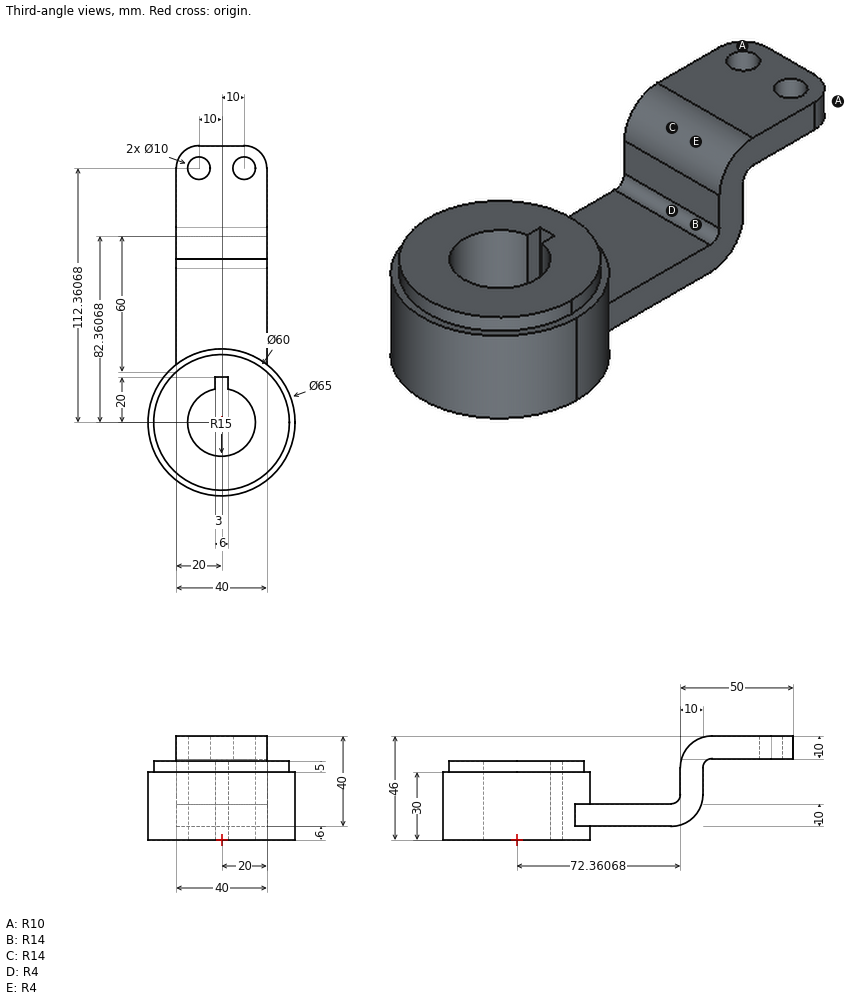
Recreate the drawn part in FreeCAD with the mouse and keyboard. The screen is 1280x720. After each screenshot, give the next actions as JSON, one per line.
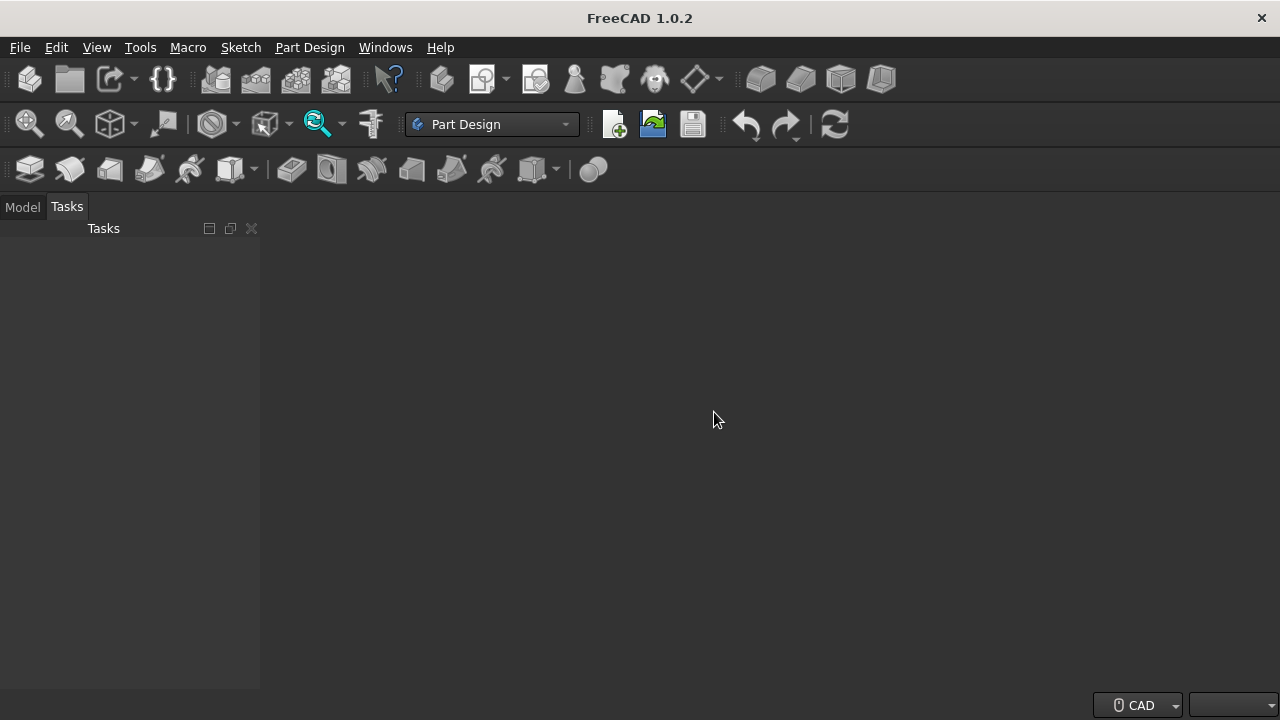
{"action": "key", "text": "ctrl+n"}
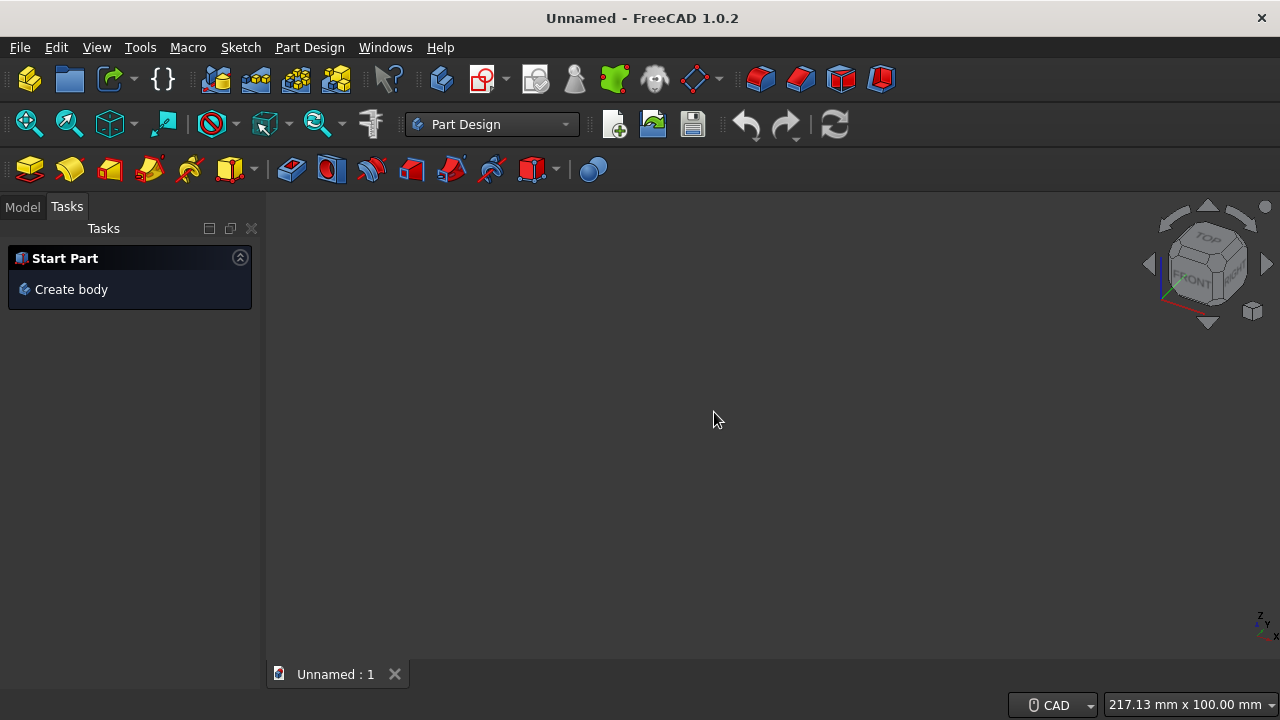
{"action": "left_click", "coordinate": [482, 80]}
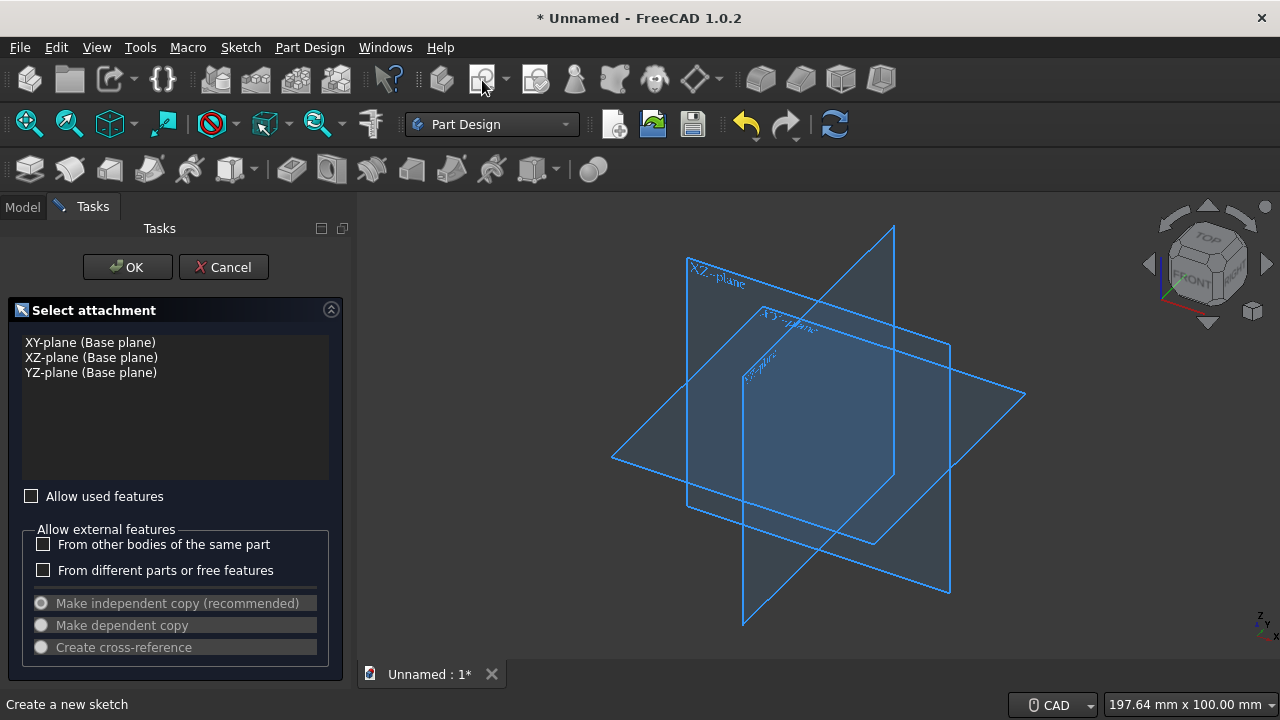
{"action": "left_click", "coordinate": [82, 342]}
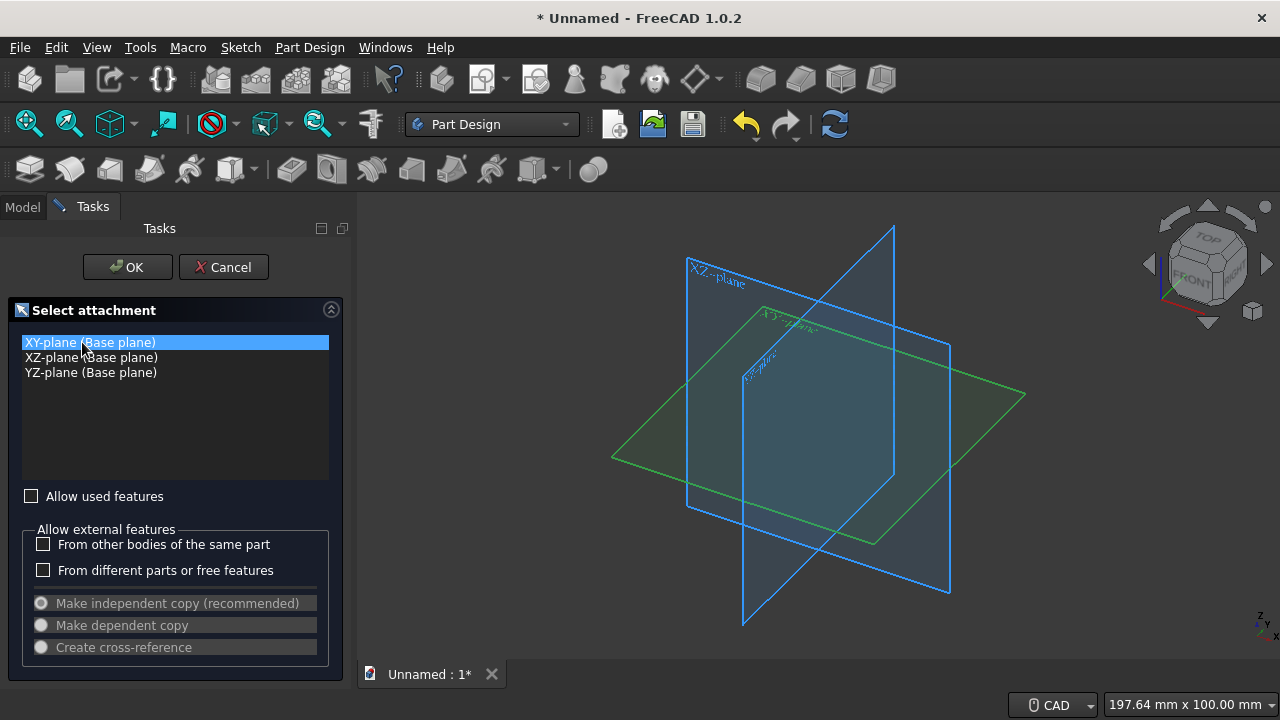
{"action": "left_click", "coordinate": [128, 267]}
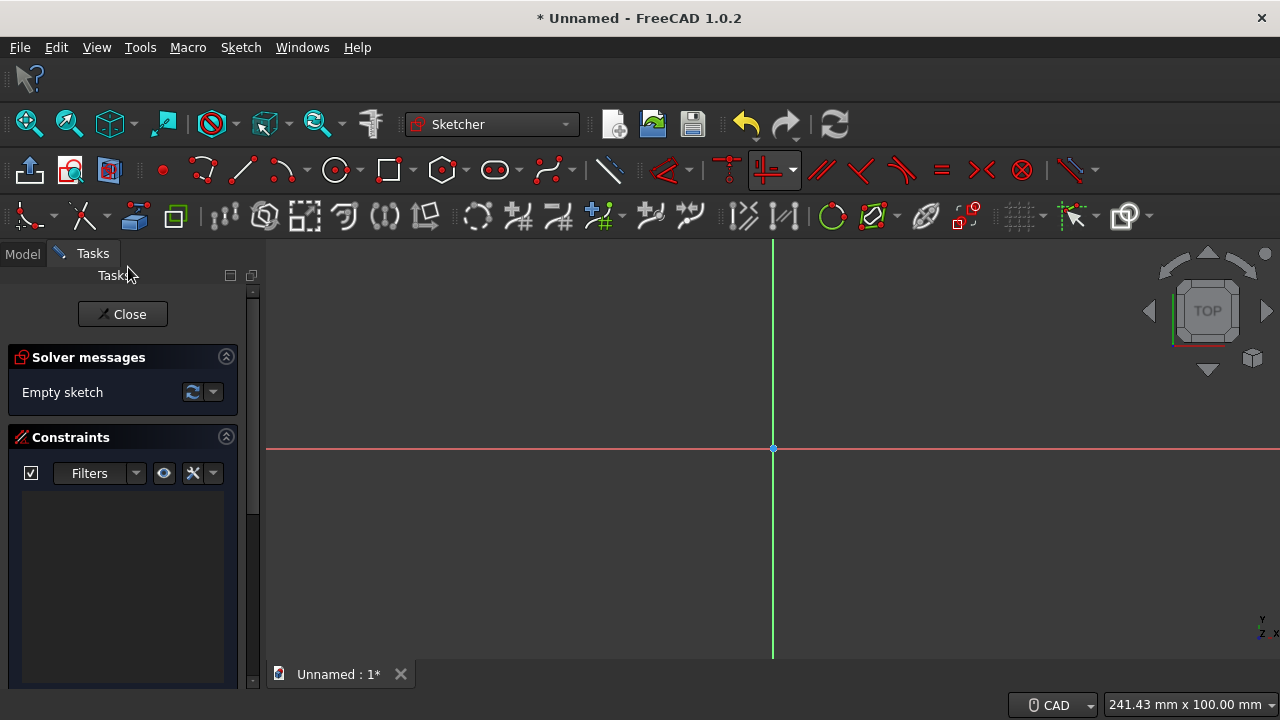
{"action": "key", "text": "g m"}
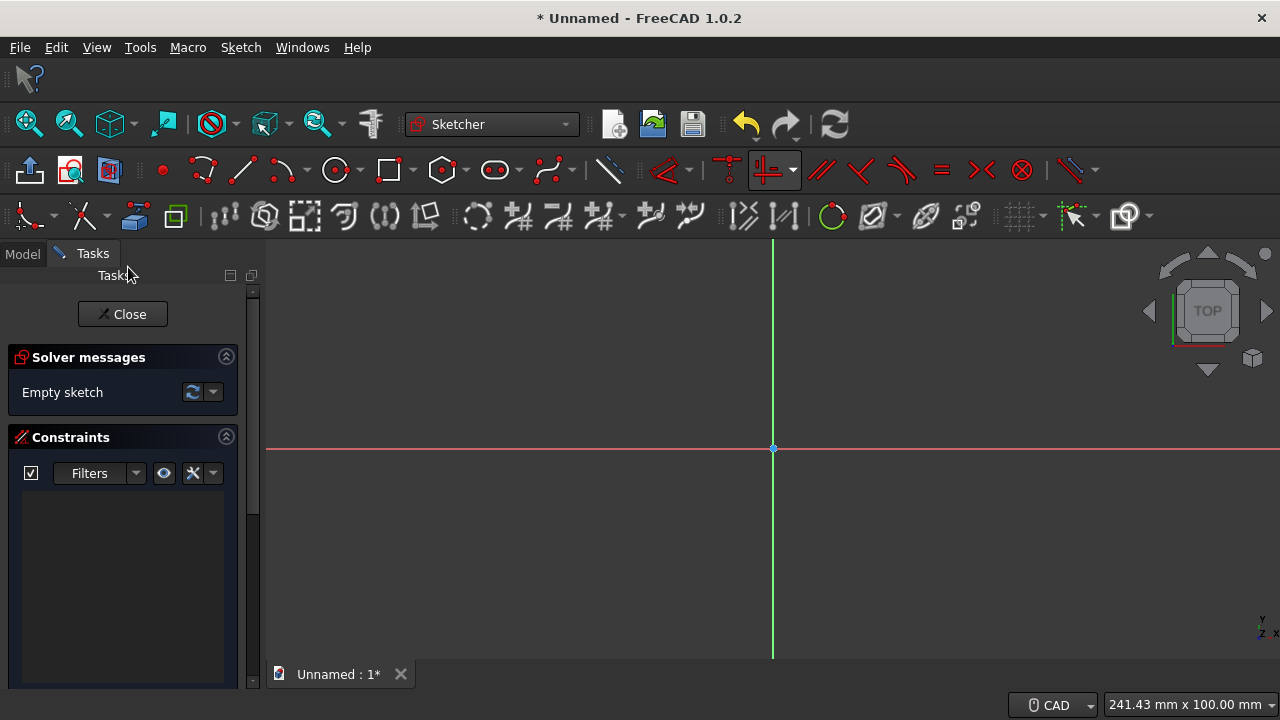
{"action": "scroll", "coordinate": [760, 387], "scroll_direction": "up", "scroll_amount": 2}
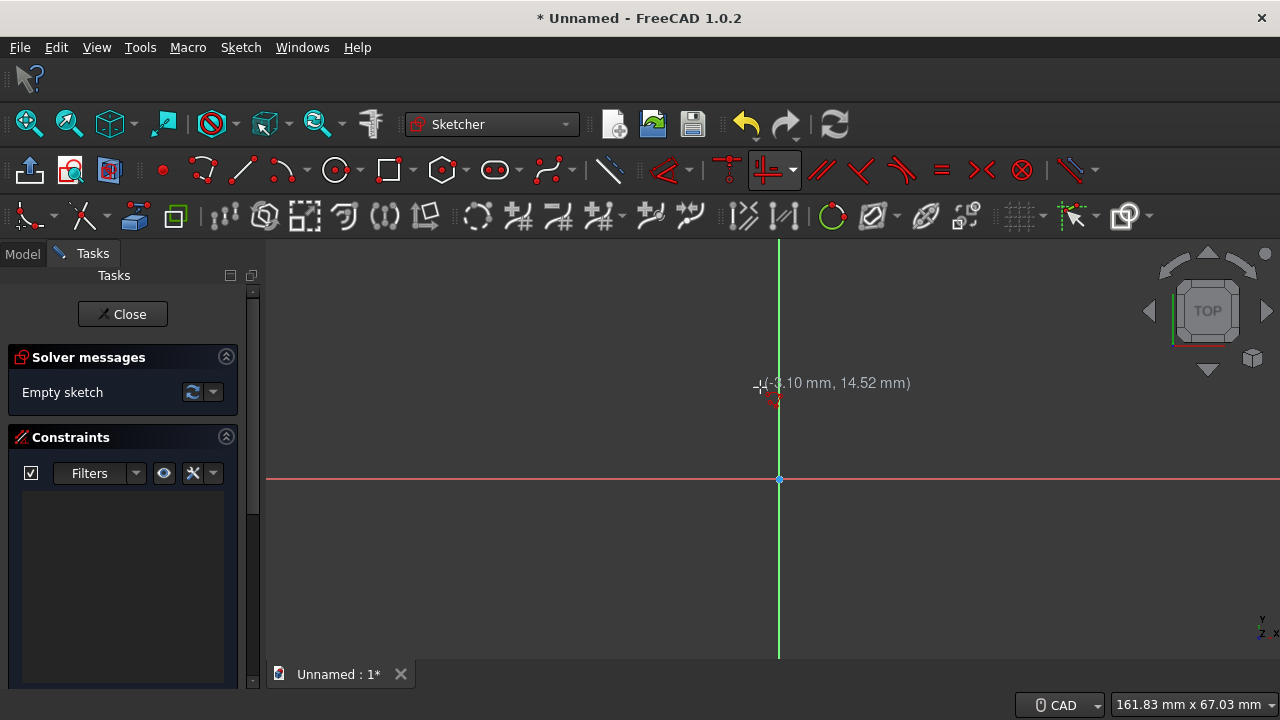
{"action": "left_click", "coordinate": [760, 387]}
{"action": "left_click", "coordinate": [760, 354]}
{"action": "left_click", "coordinate": [798, 354]}
{"action": "left_click", "coordinate": [798, 387]}
{"action": "right_click", "coordinate": [798, 387]}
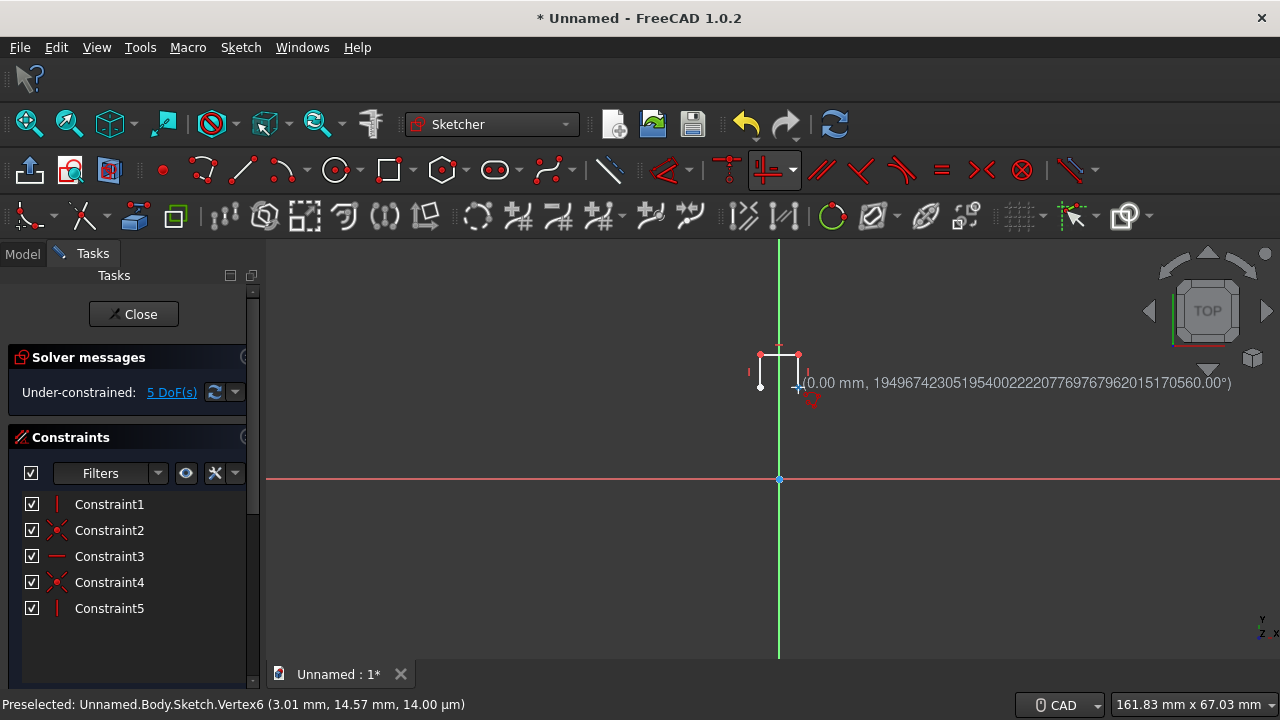
{"action": "key", "text": "g 3 a"}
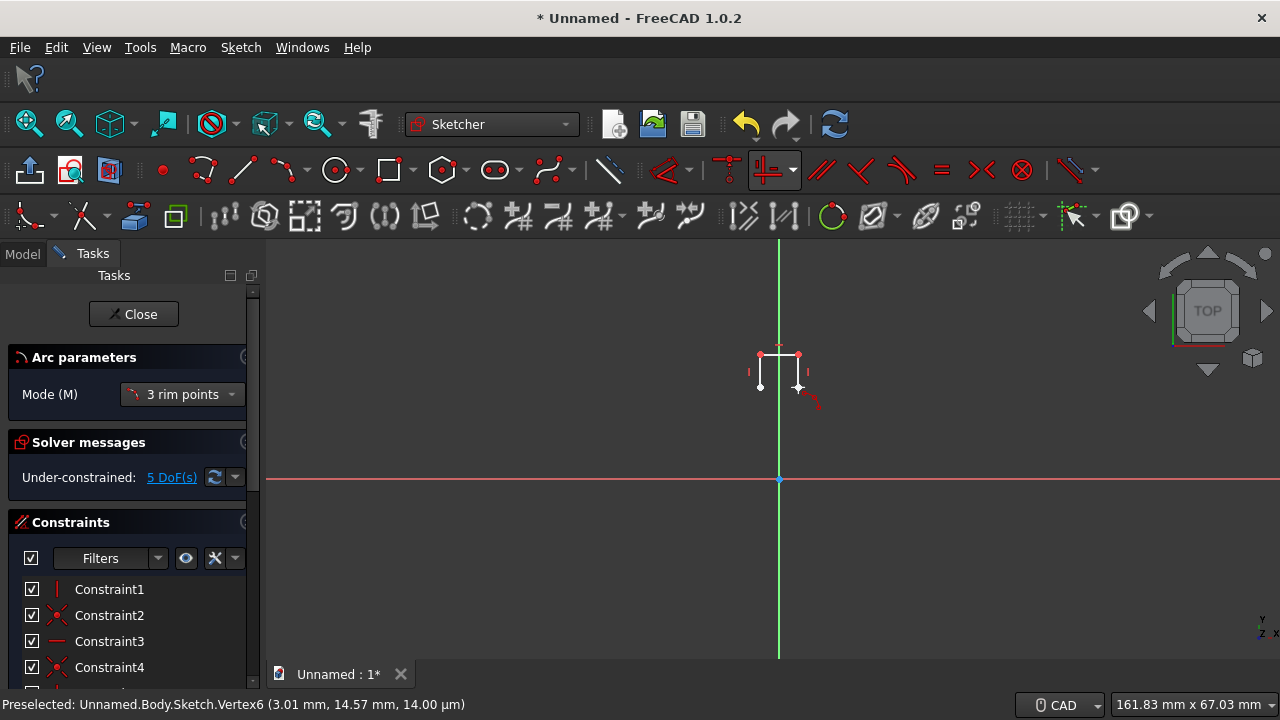
{"action": "left_click", "coordinate": [798, 388]}
{"action": "left_click", "coordinate": [760, 388]}
{"action": "left_click", "coordinate": [727, 558]}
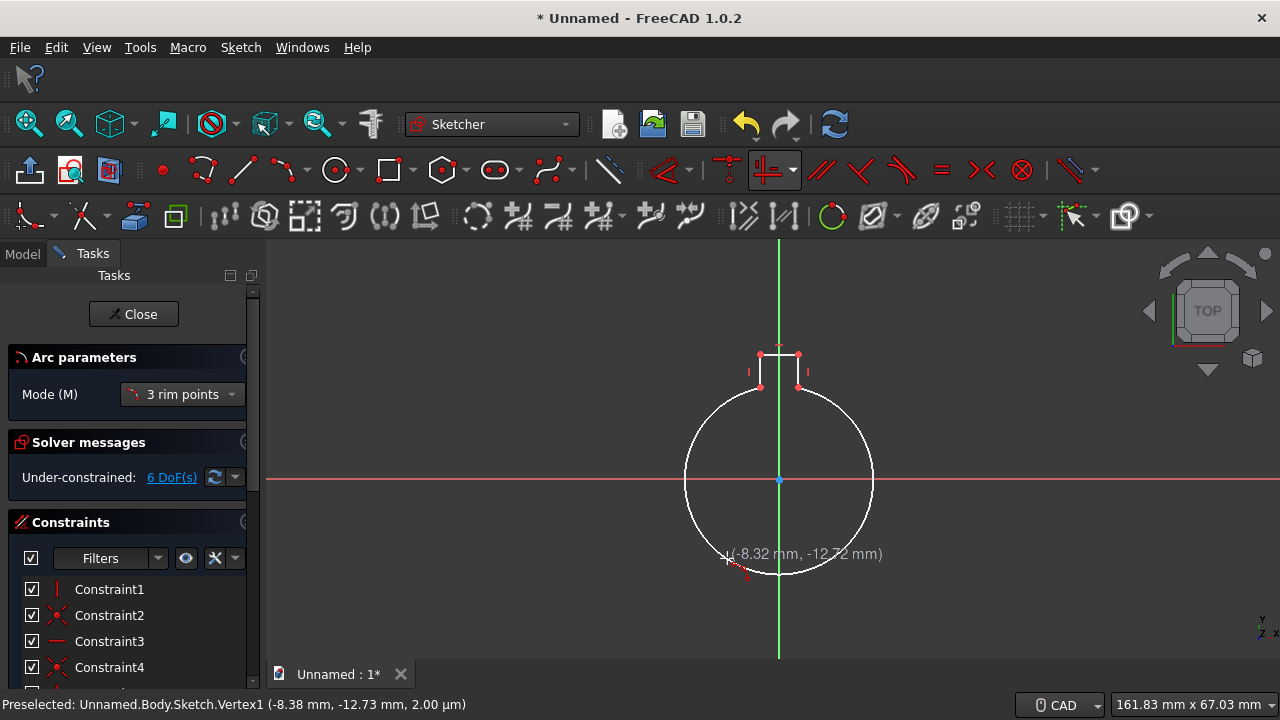
{"action": "left_click", "coordinate": [336, 170]}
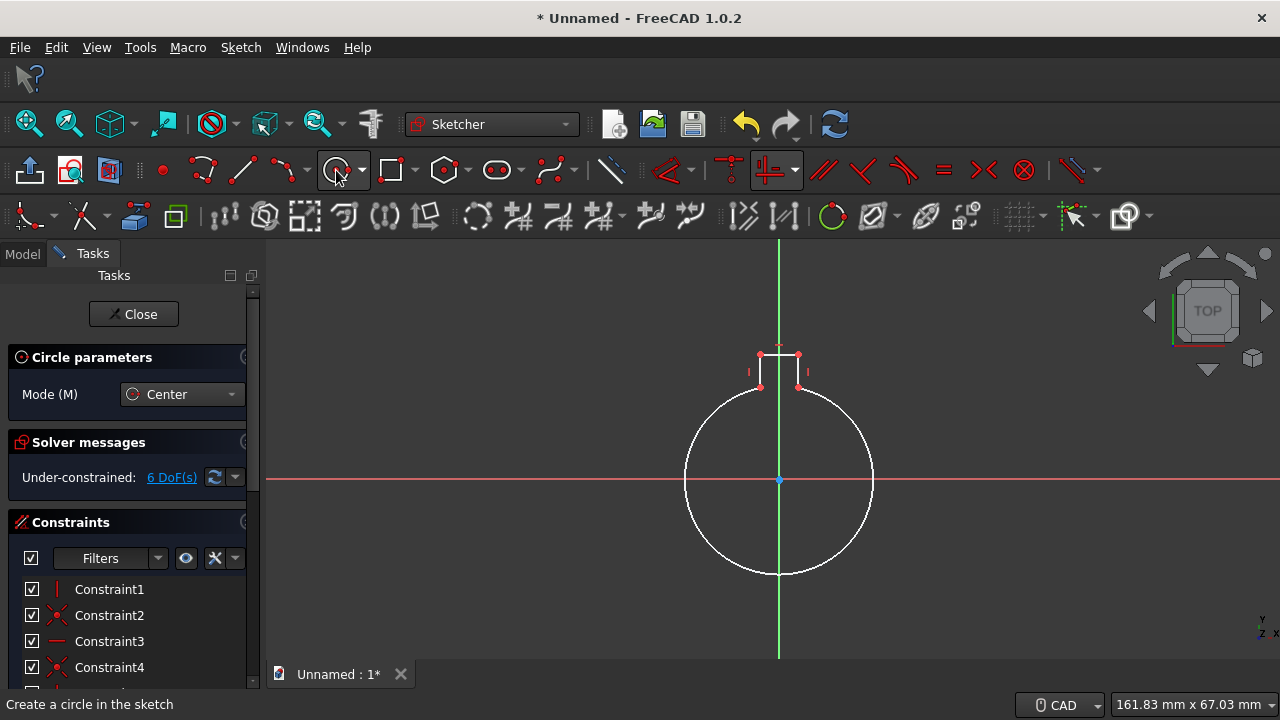
{"action": "left_click", "coordinate": [779, 479]}
{"action": "left_click", "coordinate": [923, 335]}
{"action": "key", "text": "Escape"}